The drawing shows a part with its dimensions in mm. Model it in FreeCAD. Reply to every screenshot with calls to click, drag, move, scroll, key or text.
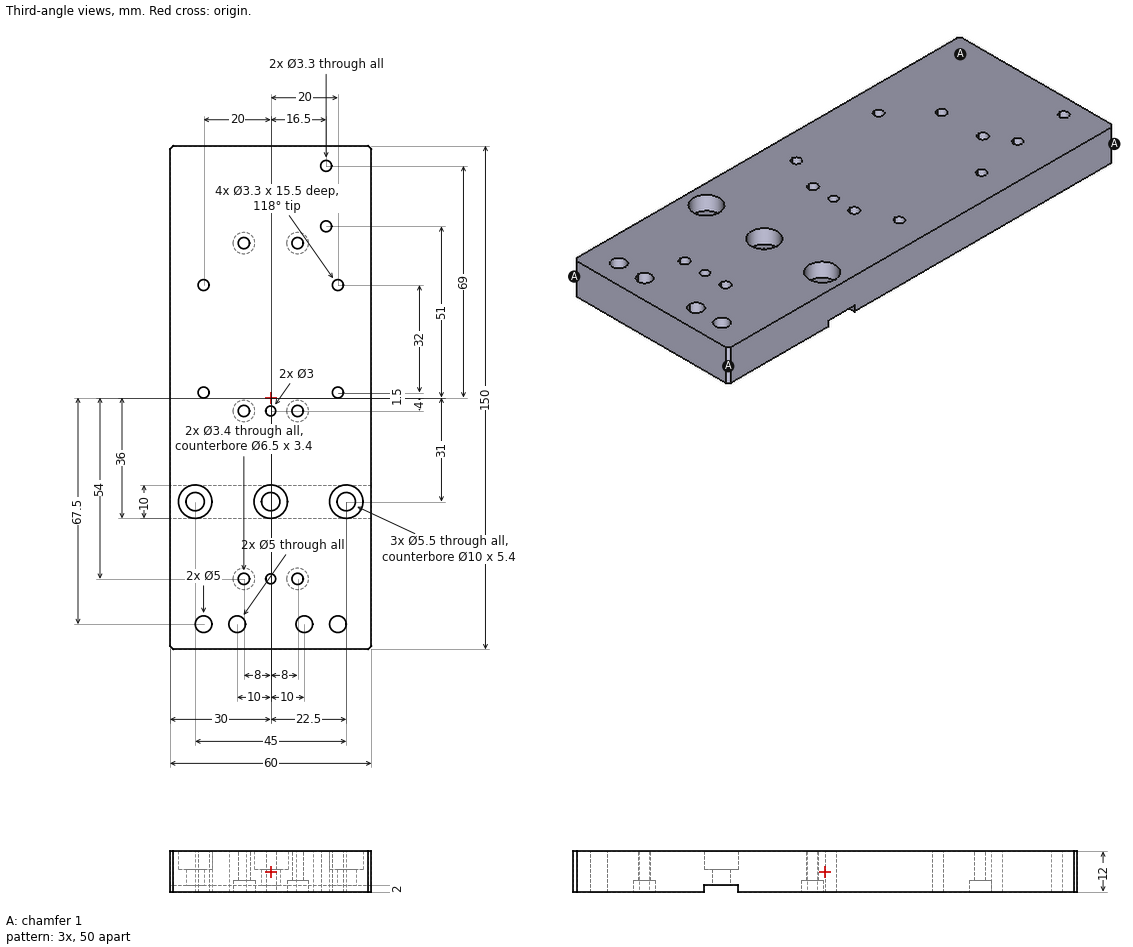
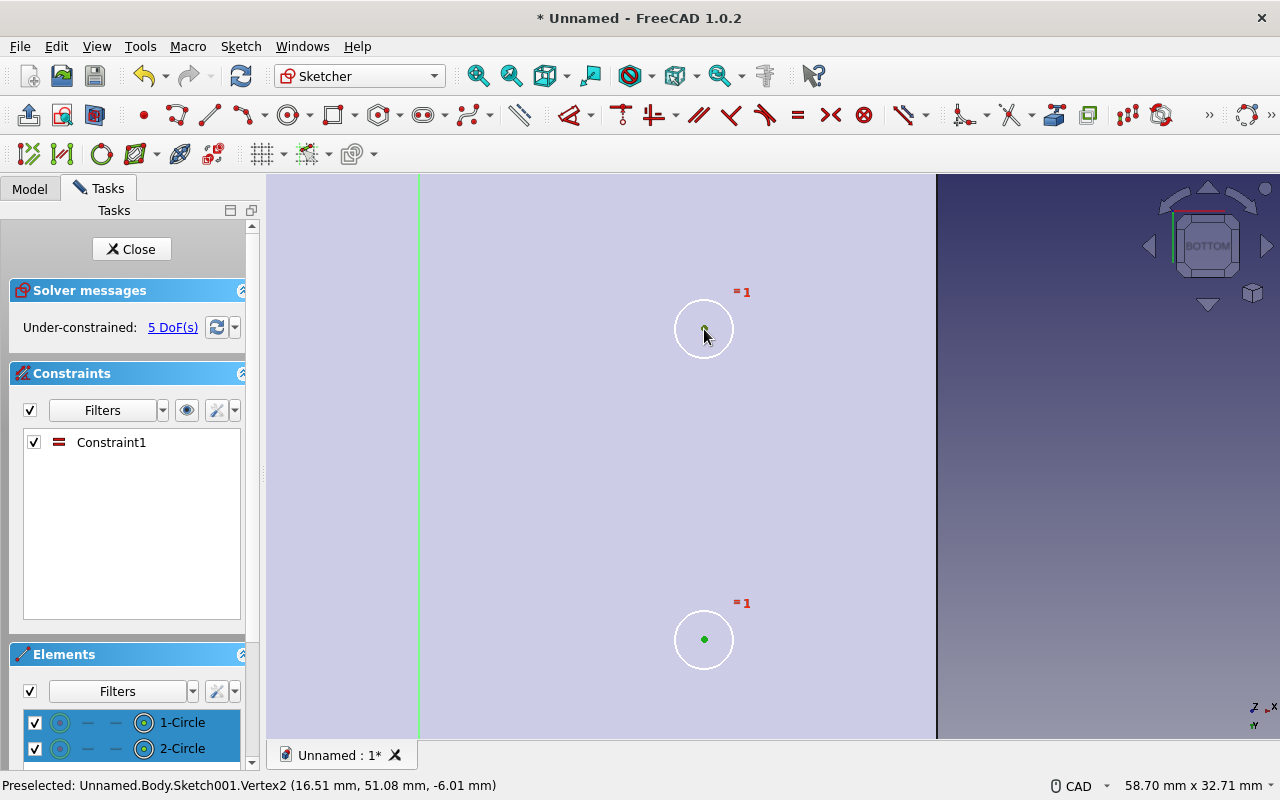
click(676, 116)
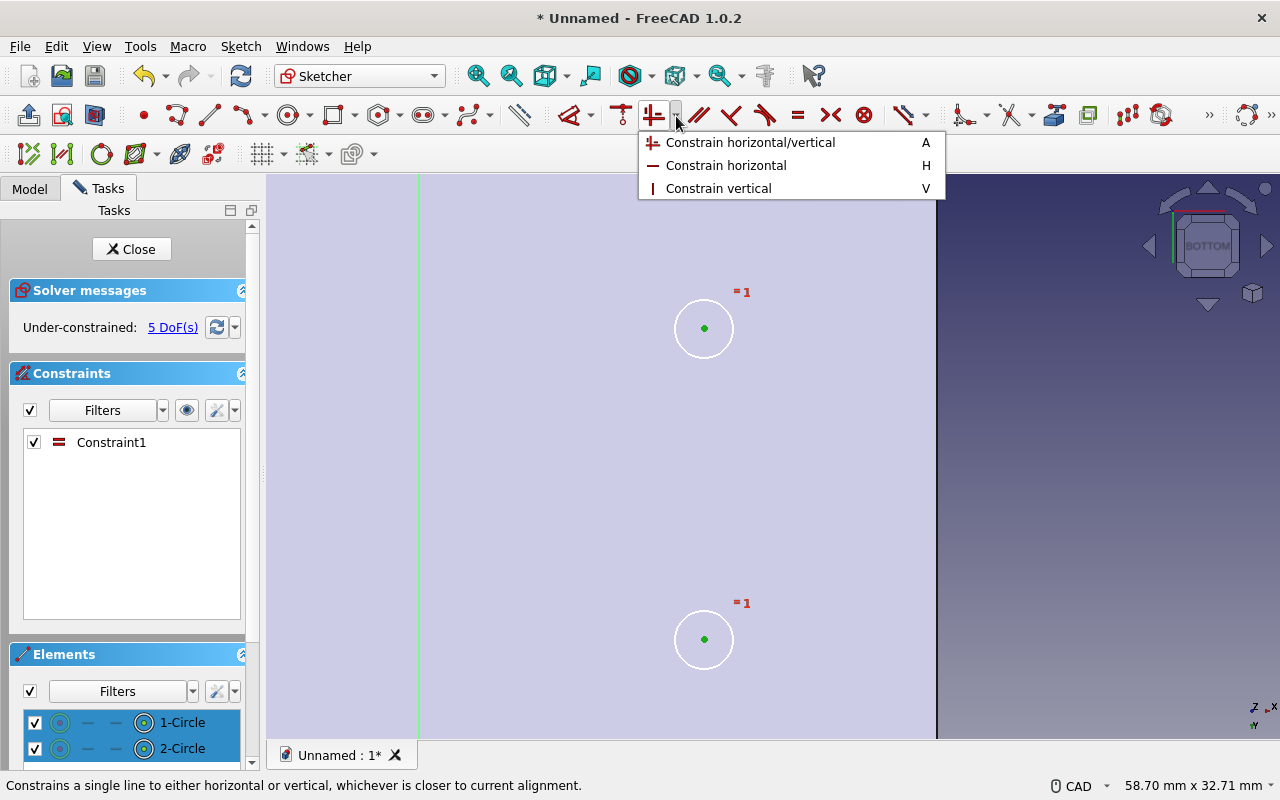
click(792, 188)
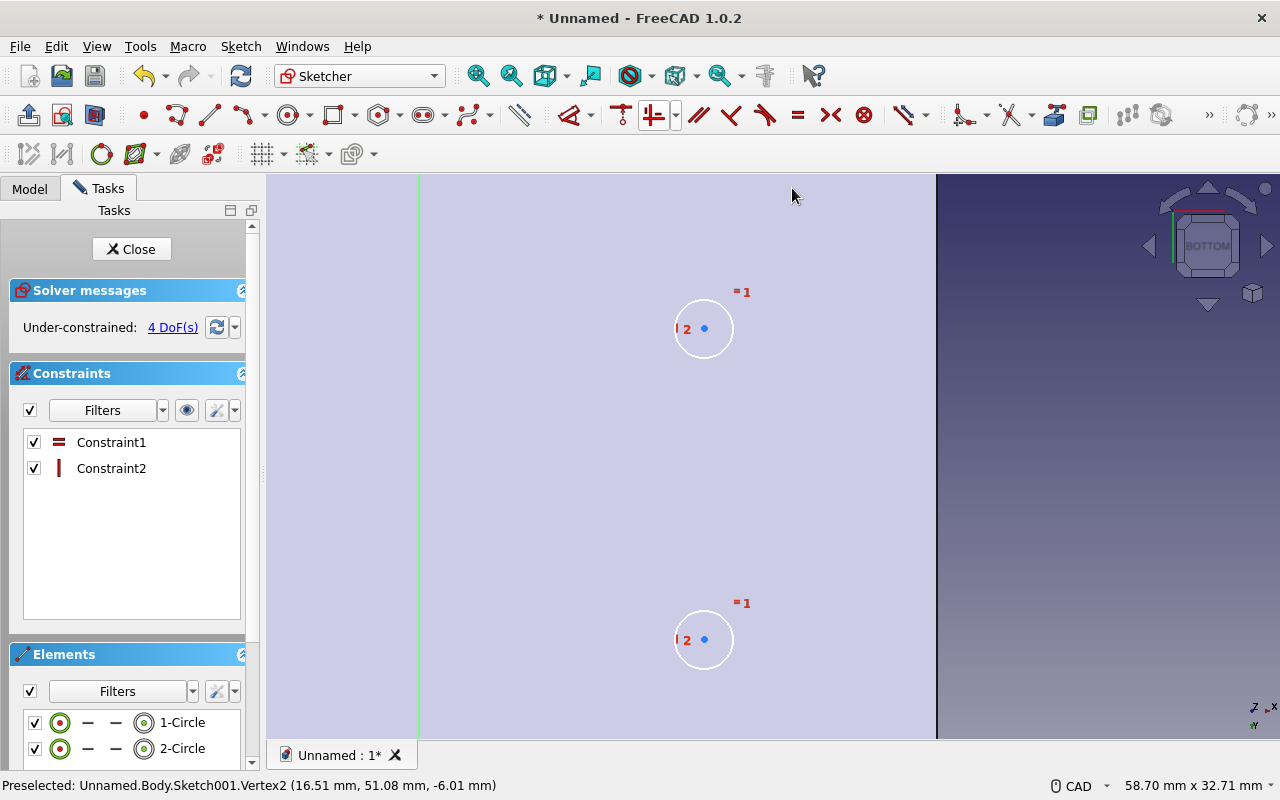
click(568, 116)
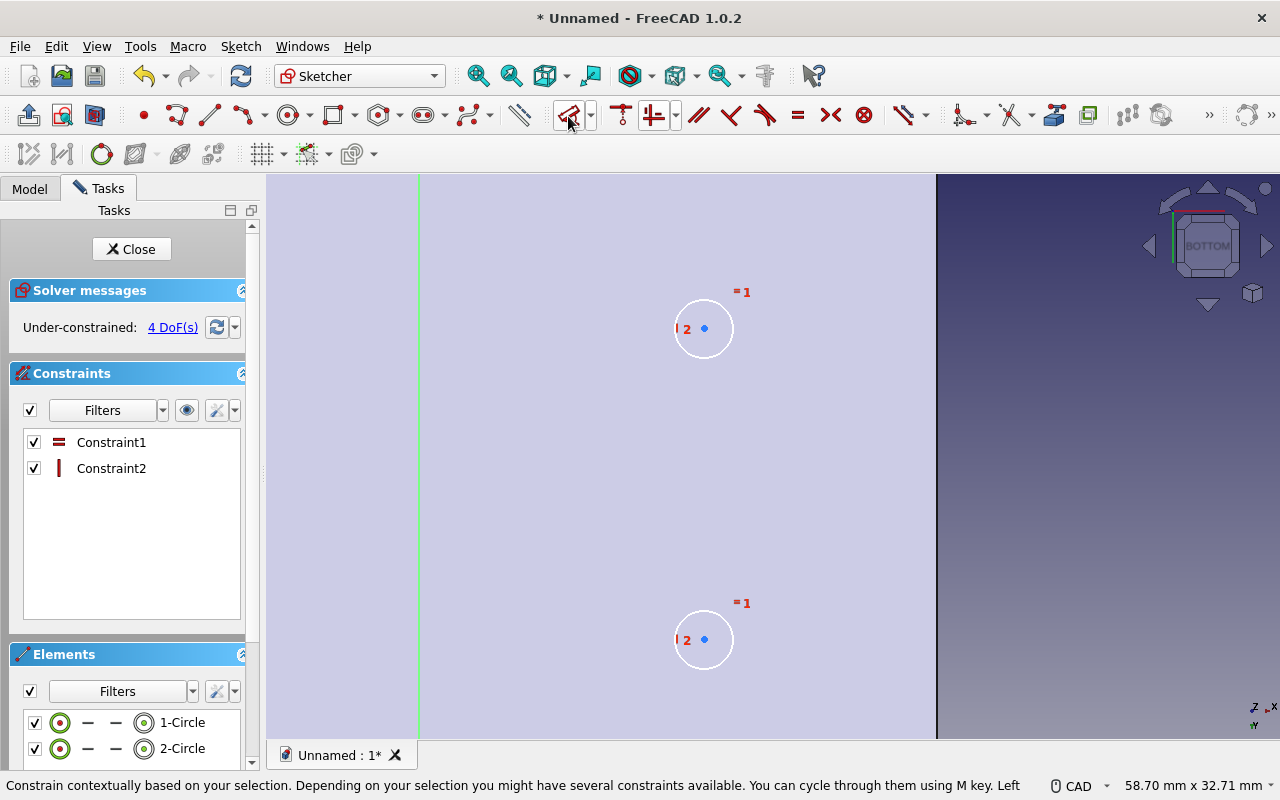
click(724, 619)
click(746, 596)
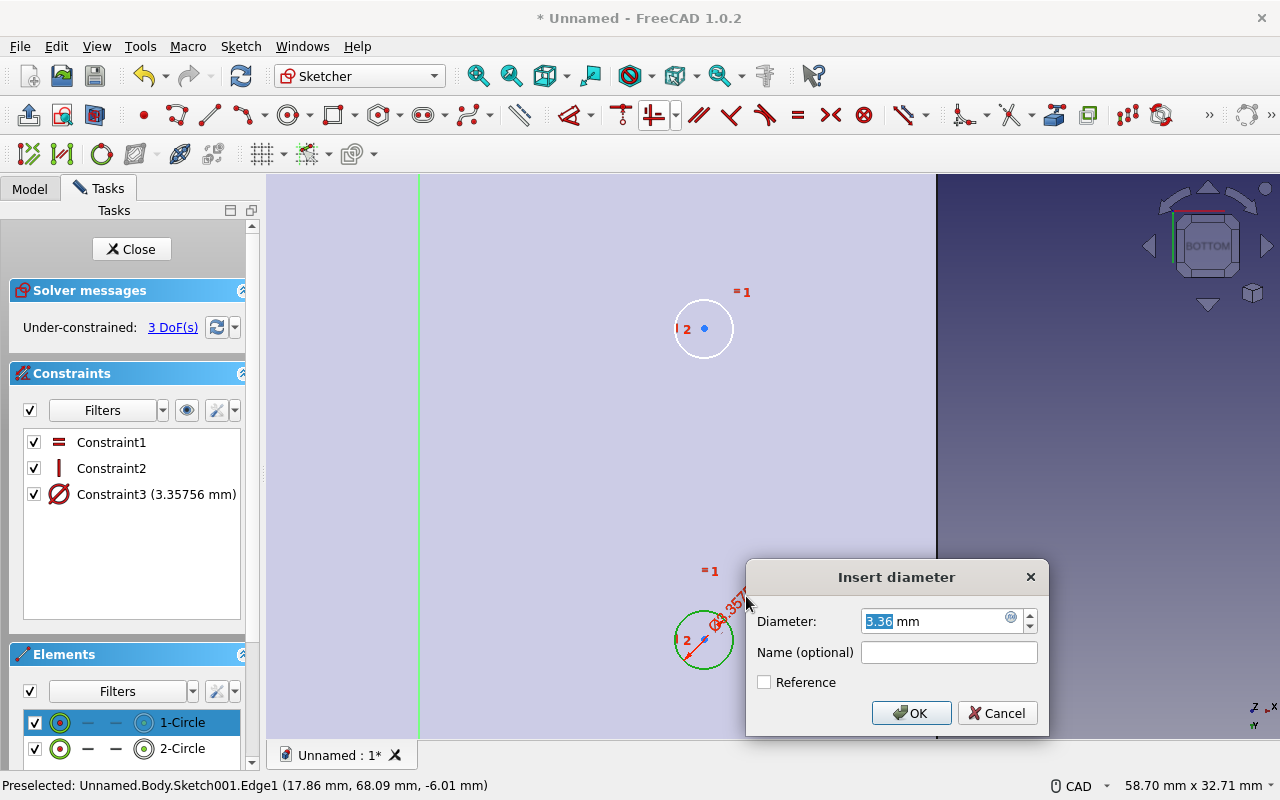
text(3.3)
key(Return)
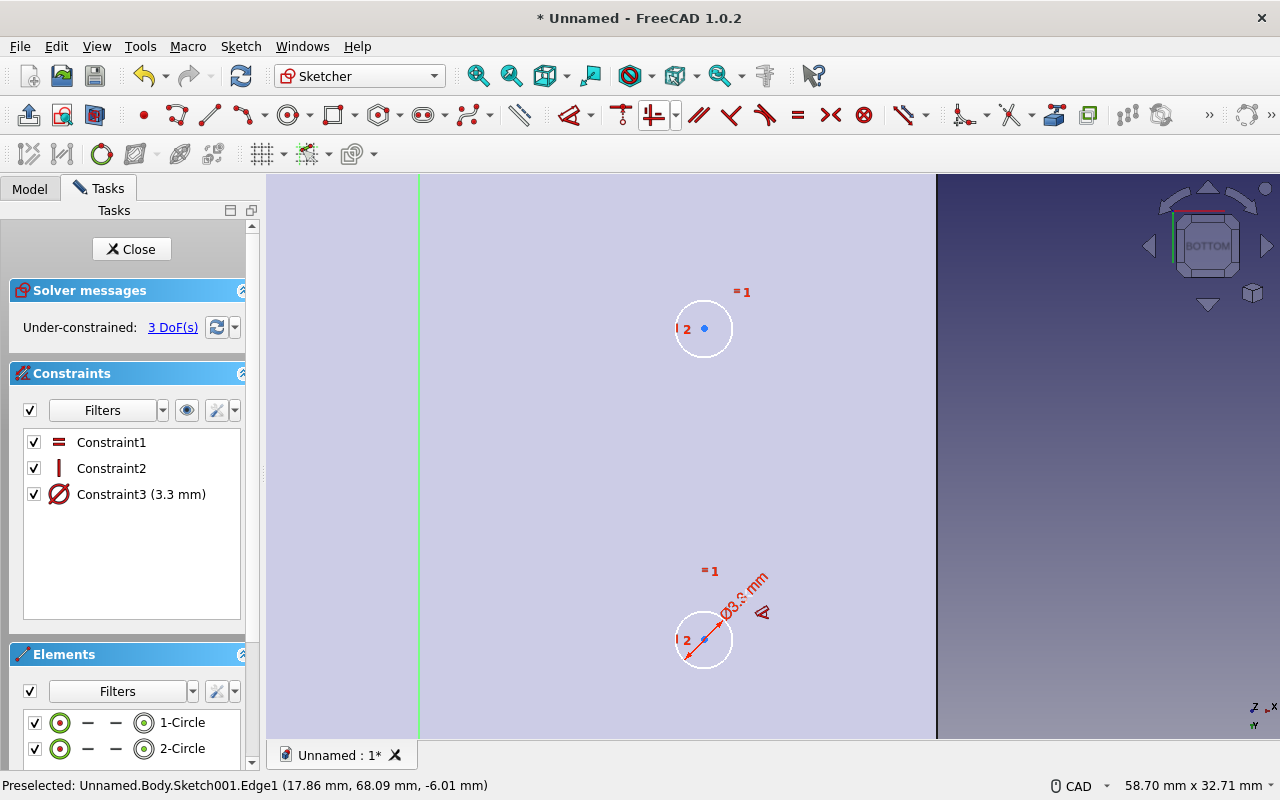
click(704, 640)
click(385, 421)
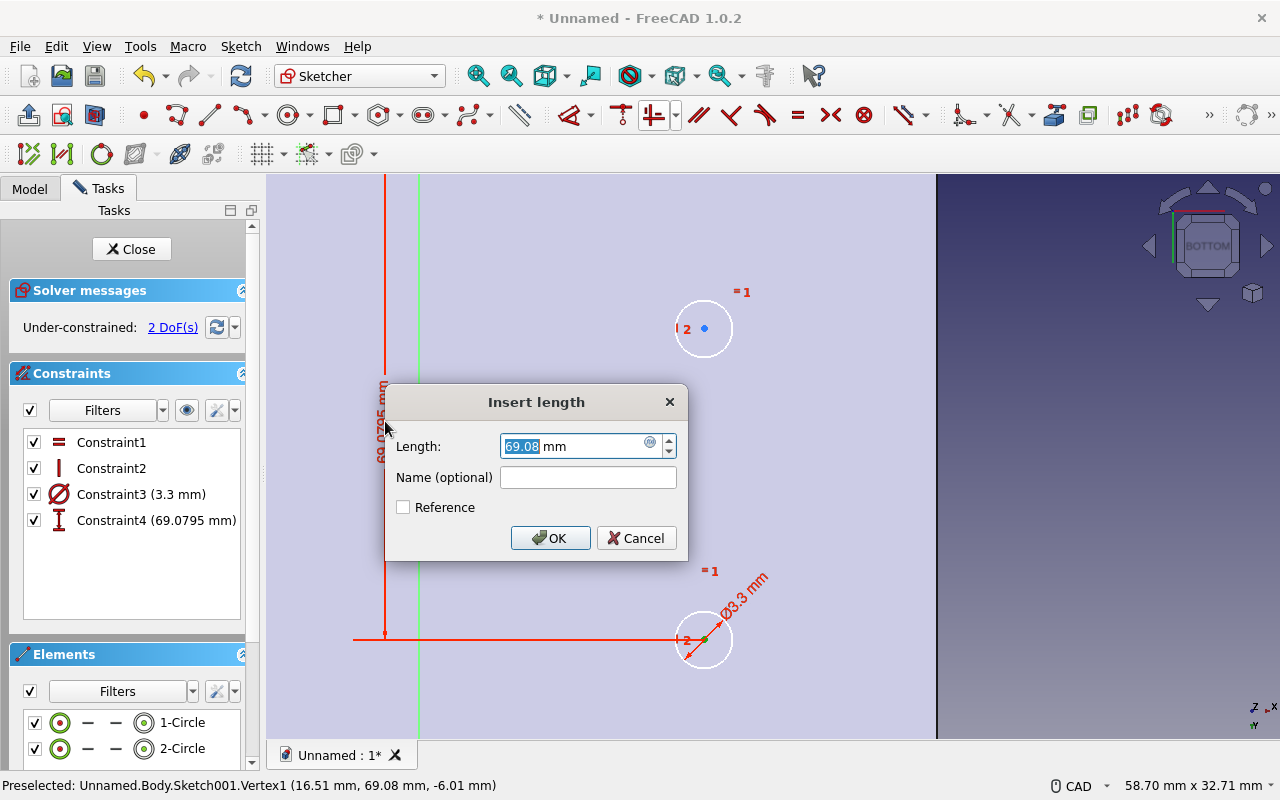
text(69)
key(Return)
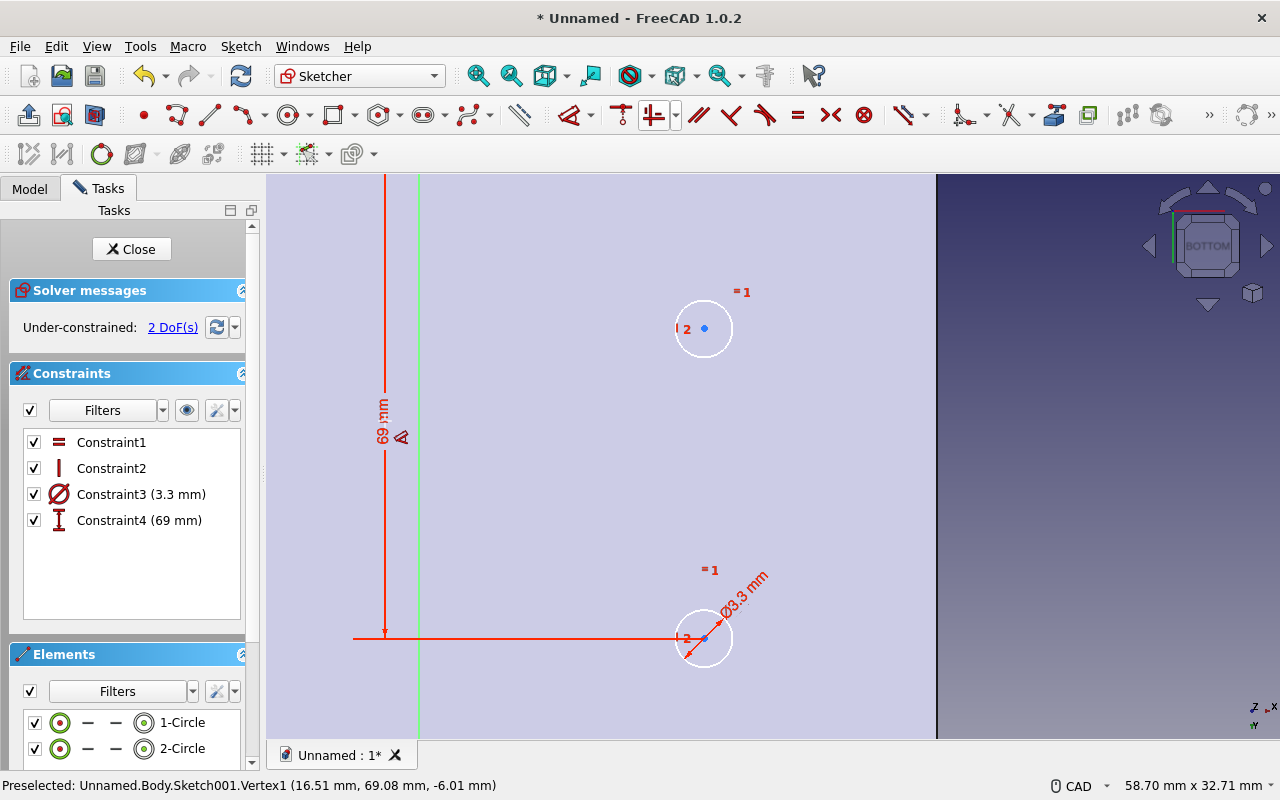
click(704, 329)
click(385, 266)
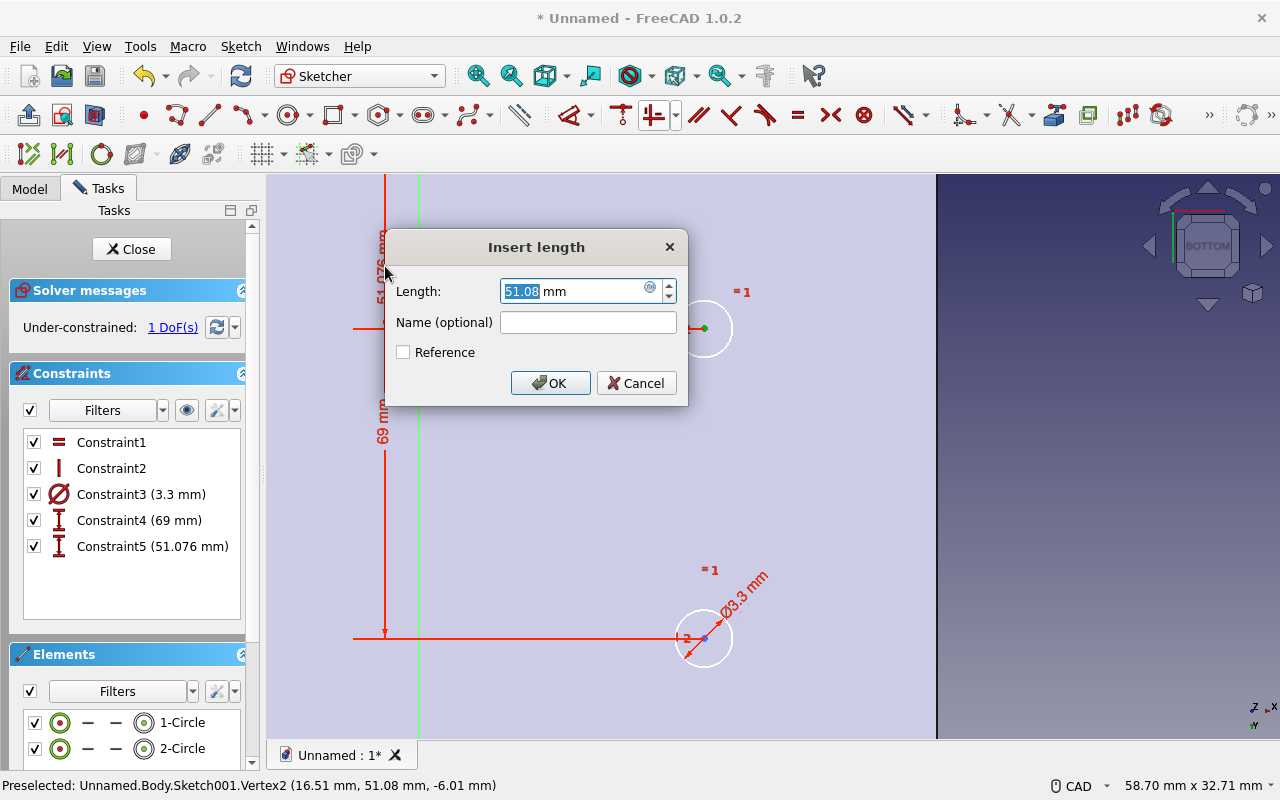
text(51)
key(Return)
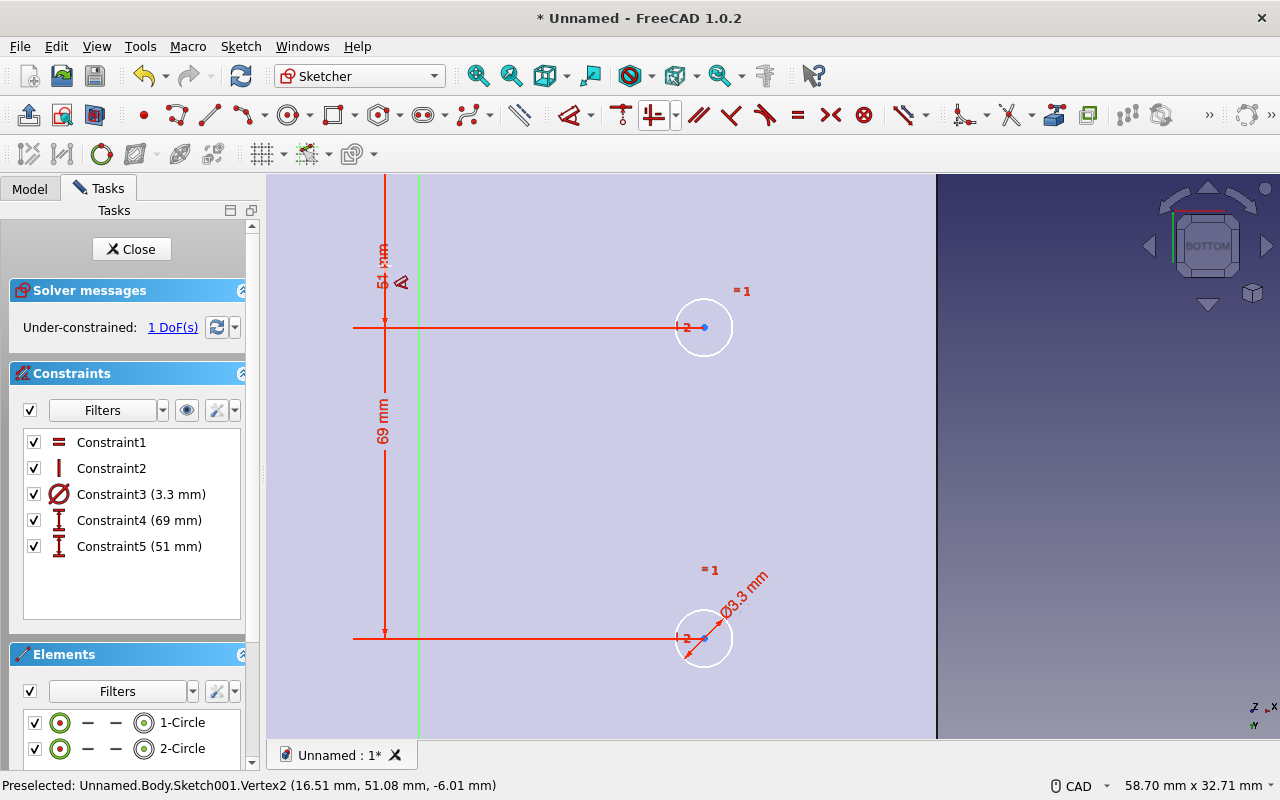
click(704, 639)
click(561, 673)